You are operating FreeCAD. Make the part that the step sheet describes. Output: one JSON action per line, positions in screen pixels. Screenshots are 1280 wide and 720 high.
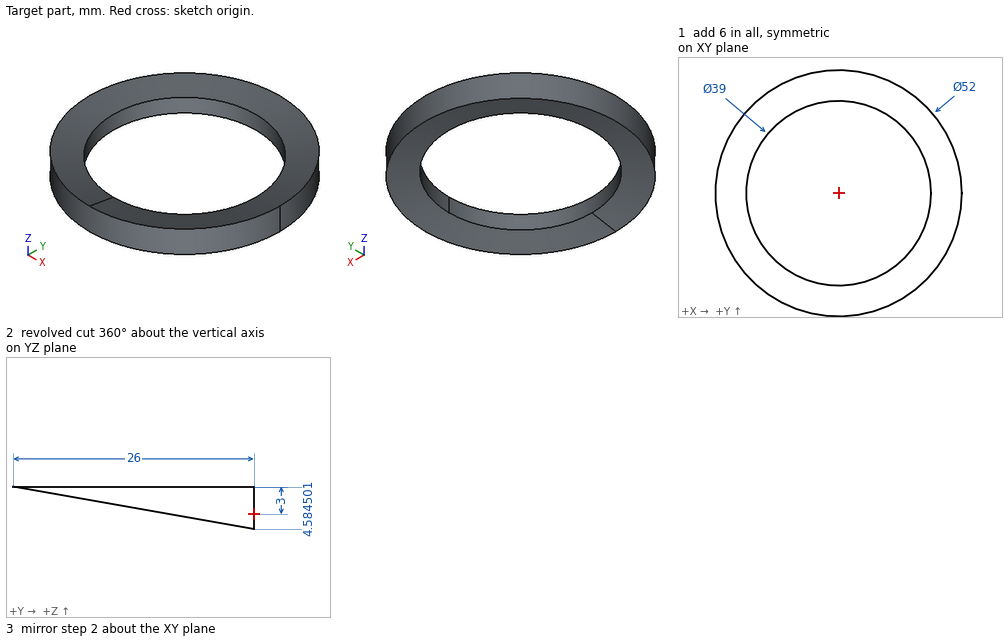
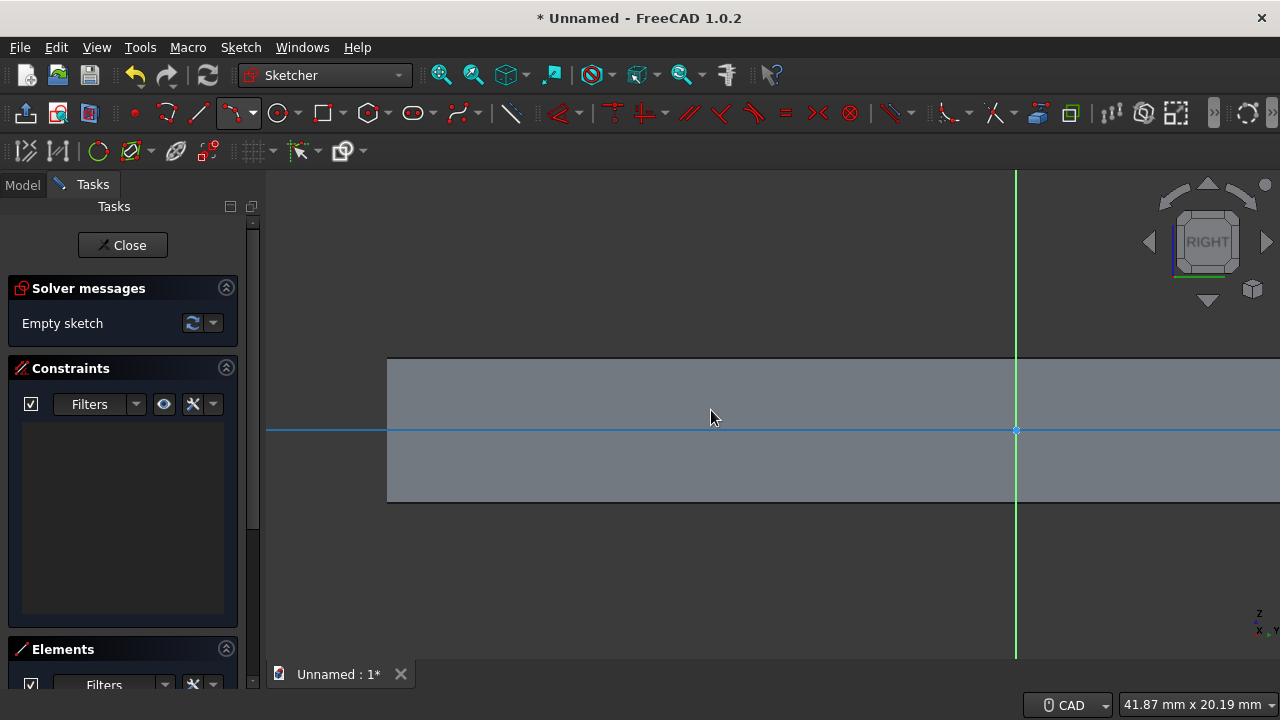
{"action": "key", "text": "g m"}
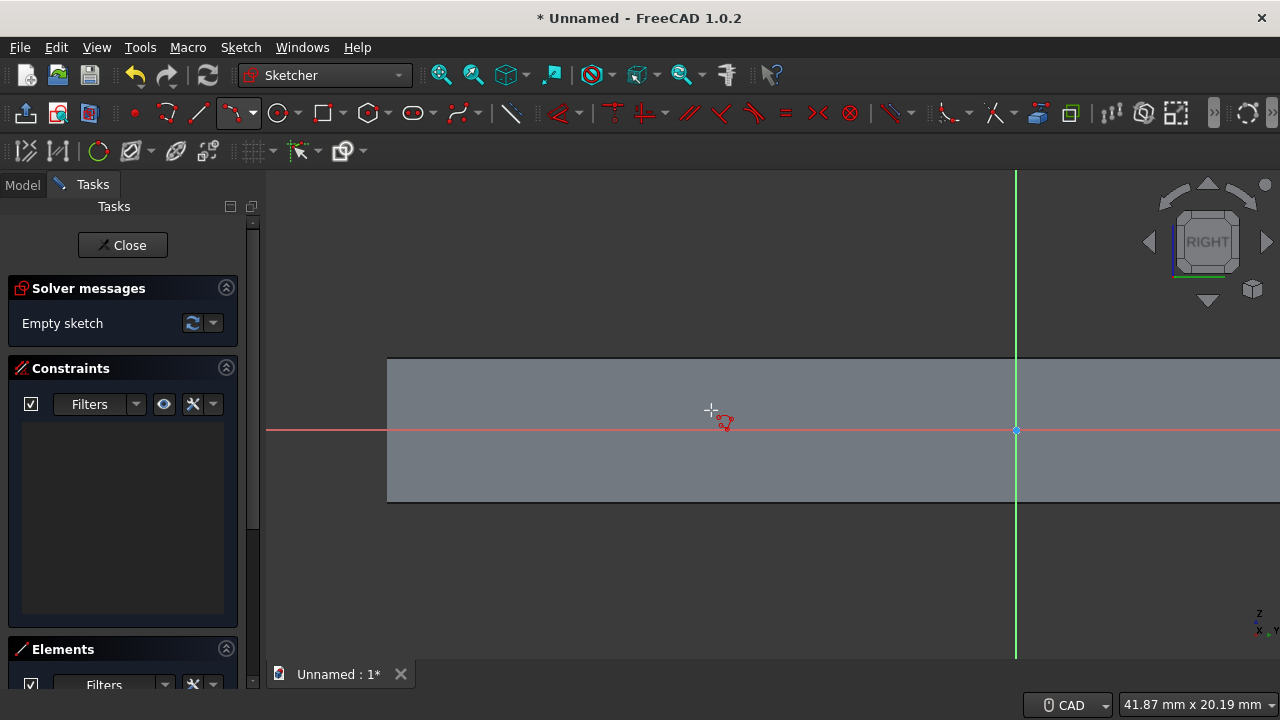
{"action": "left_click", "coordinate": [1016, 469]}
{"action": "left_click", "coordinate": [1007, 358]}
{"action": "left_click", "coordinate": [387, 358]}
{"action": "left_click", "coordinate": [1016, 470]}
{"action": "key", "text": "Escape"}
{"action": "key", "text": "Escape"}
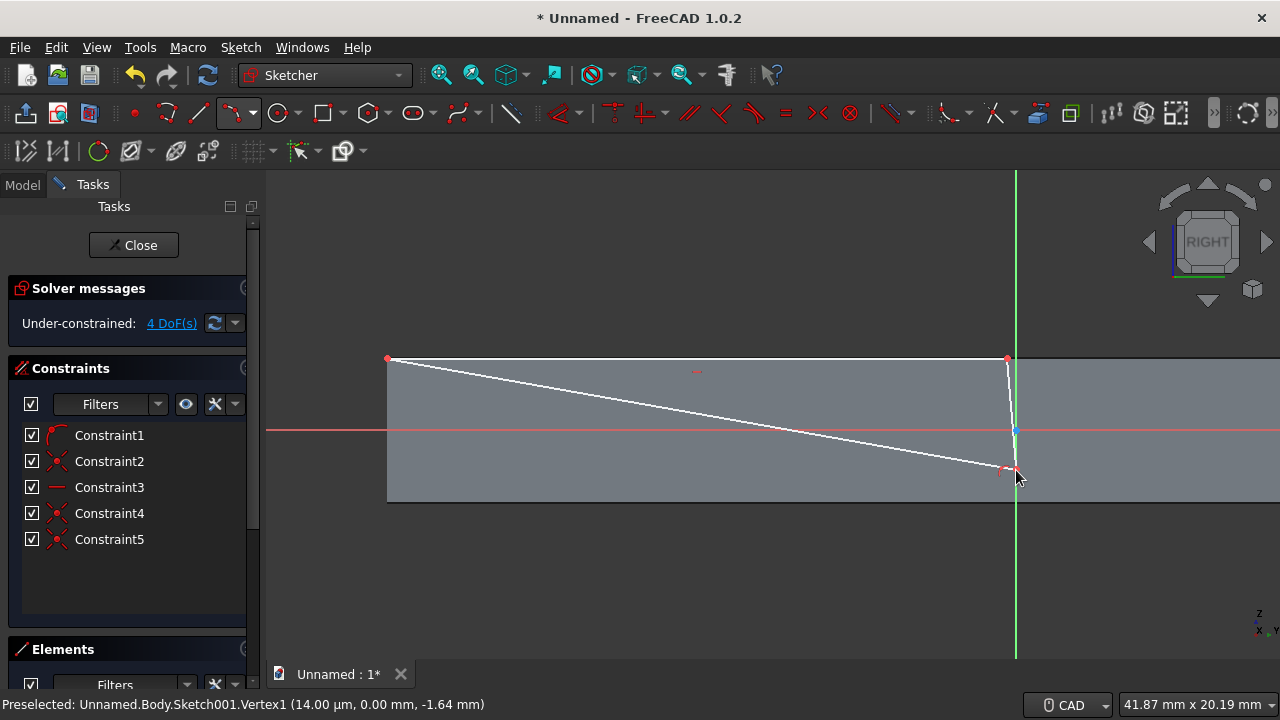
{"action": "left_click", "coordinate": [1014, 448]}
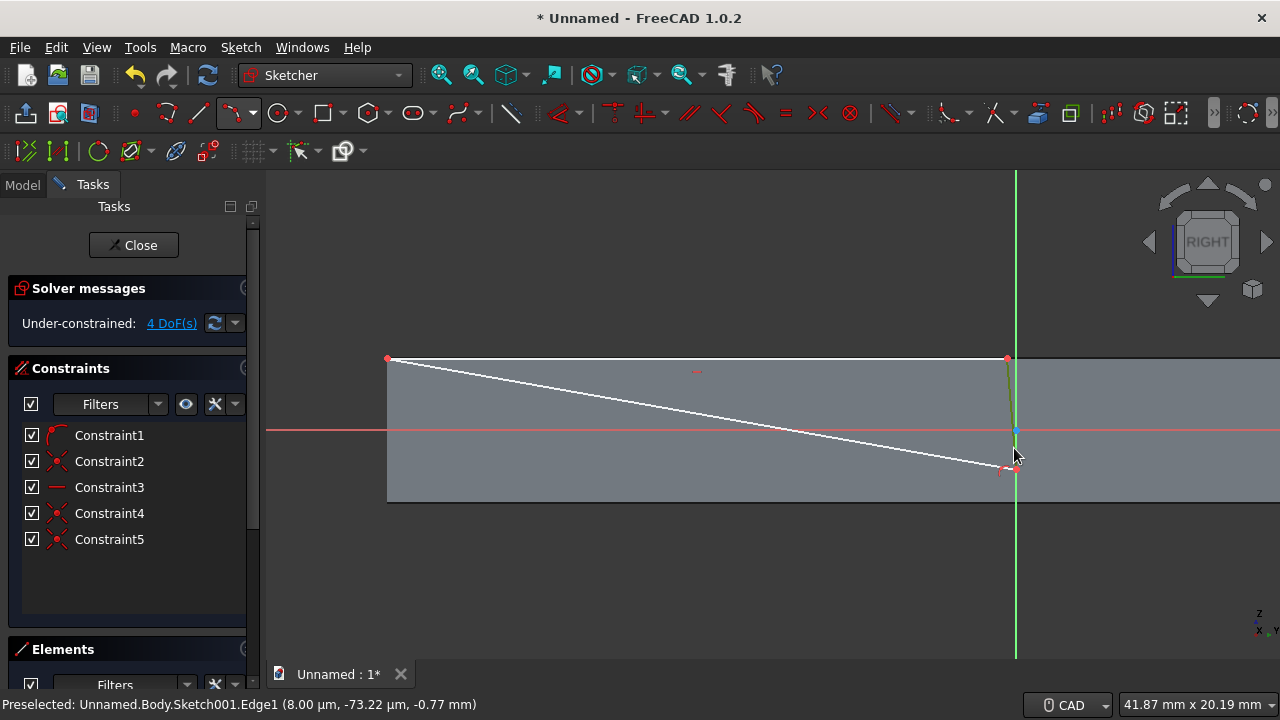
{"action": "key", "text": "v"}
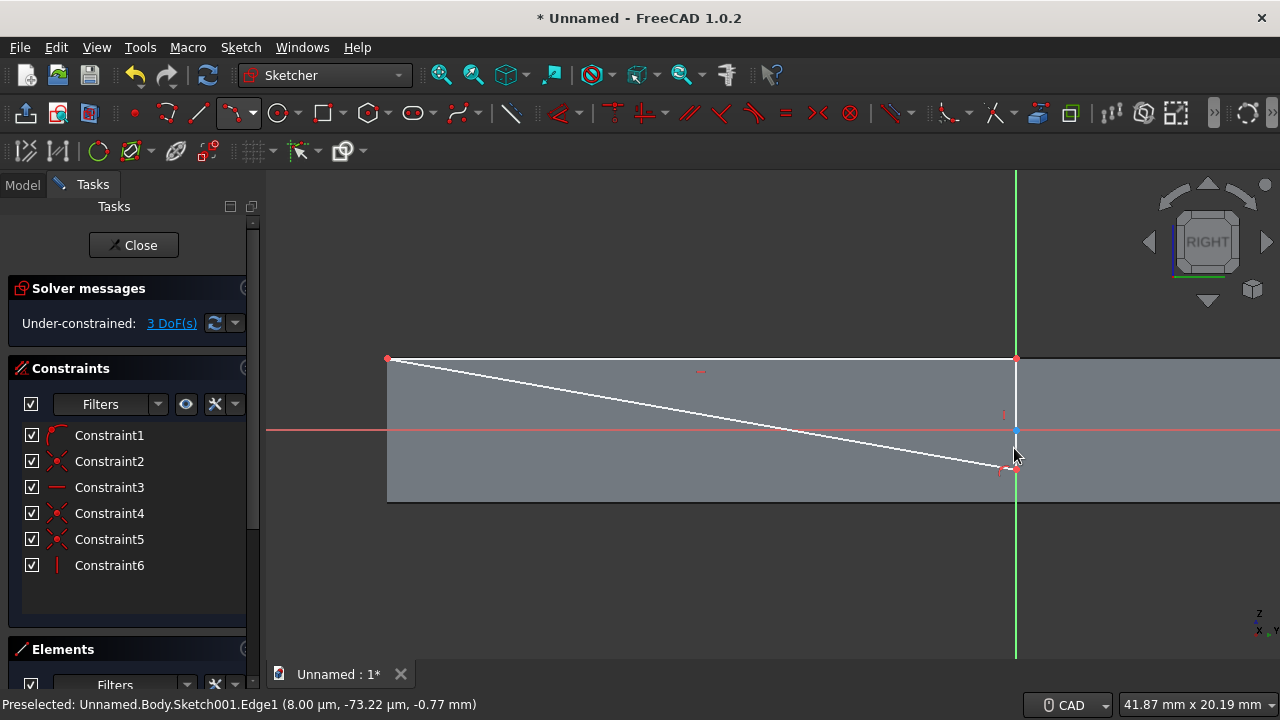
{"action": "left_click", "coordinate": [558, 114]}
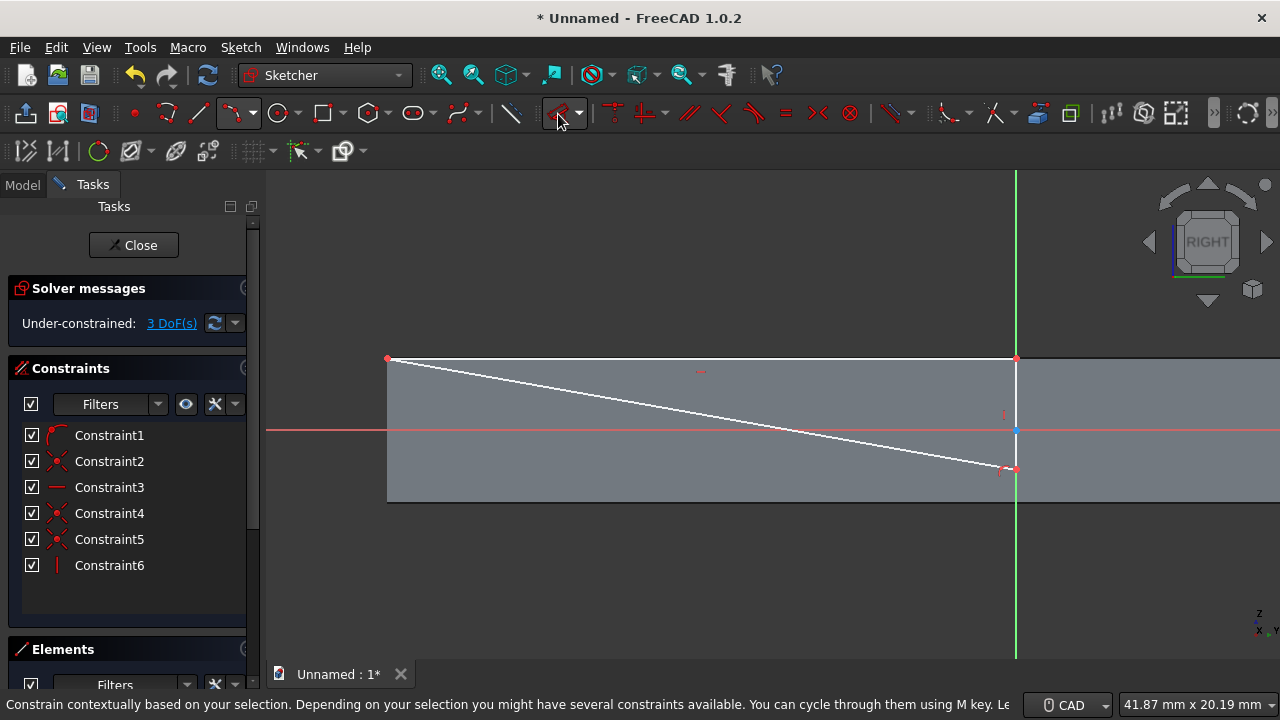
{"action": "left_click", "coordinate": [828, 359]}
{"action": "left_click", "coordinate": [702, 325]}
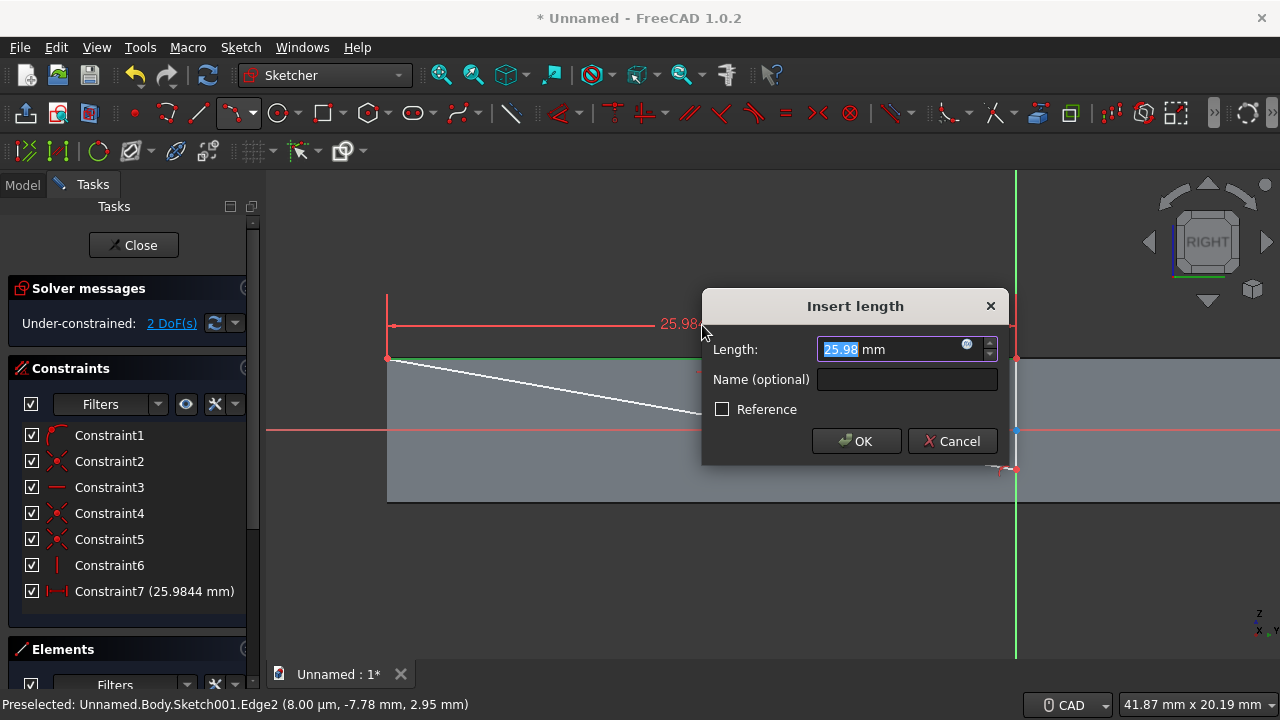
{"action": "type", "text": "26"}
{"action": "key", "text": "Return"}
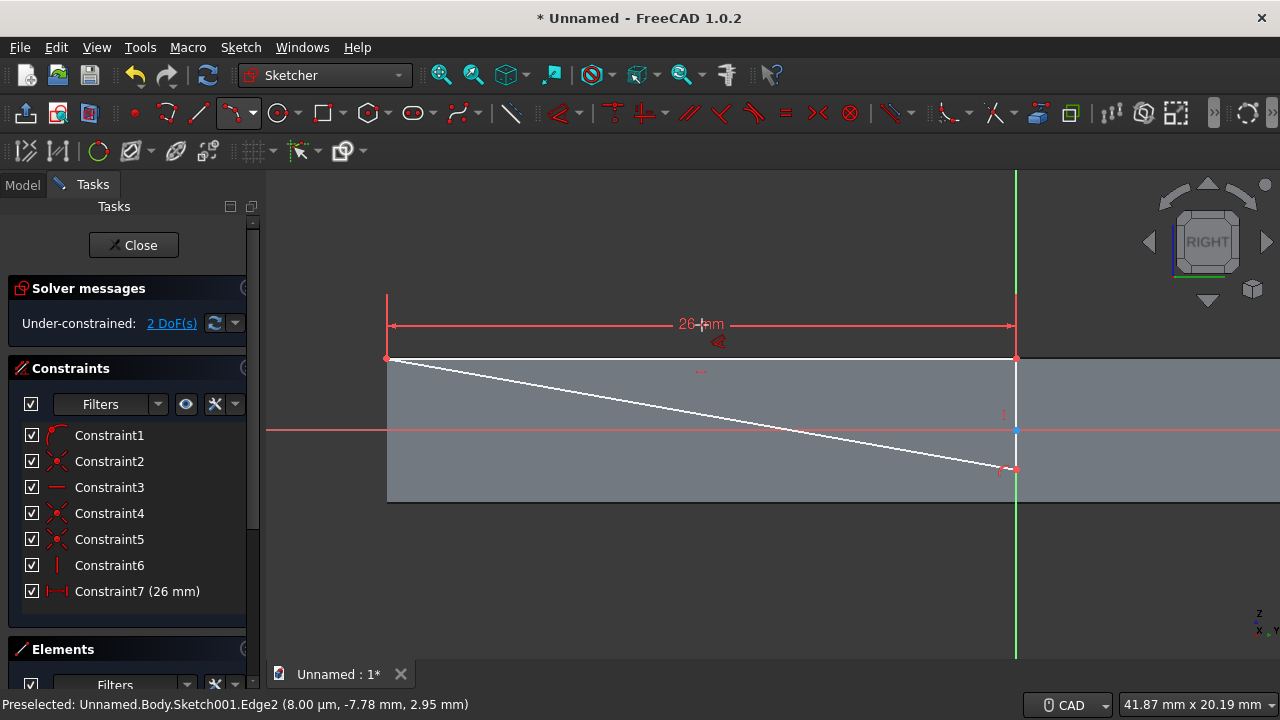
{"action": "left_click", "coordinate": [1016, 359]}
{"action": "left_click", "coordinate": [1050, 395]}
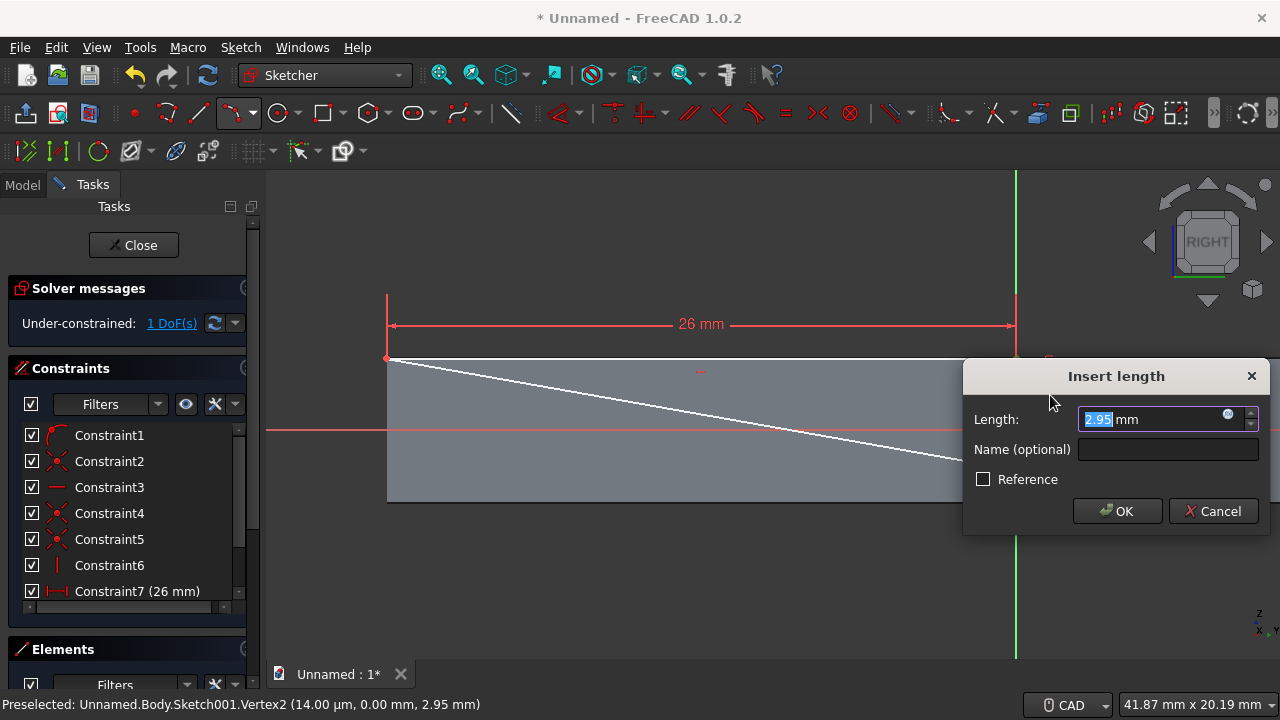
{"action": "type", "text": "3"}
{"action": "key", "text": "Return"}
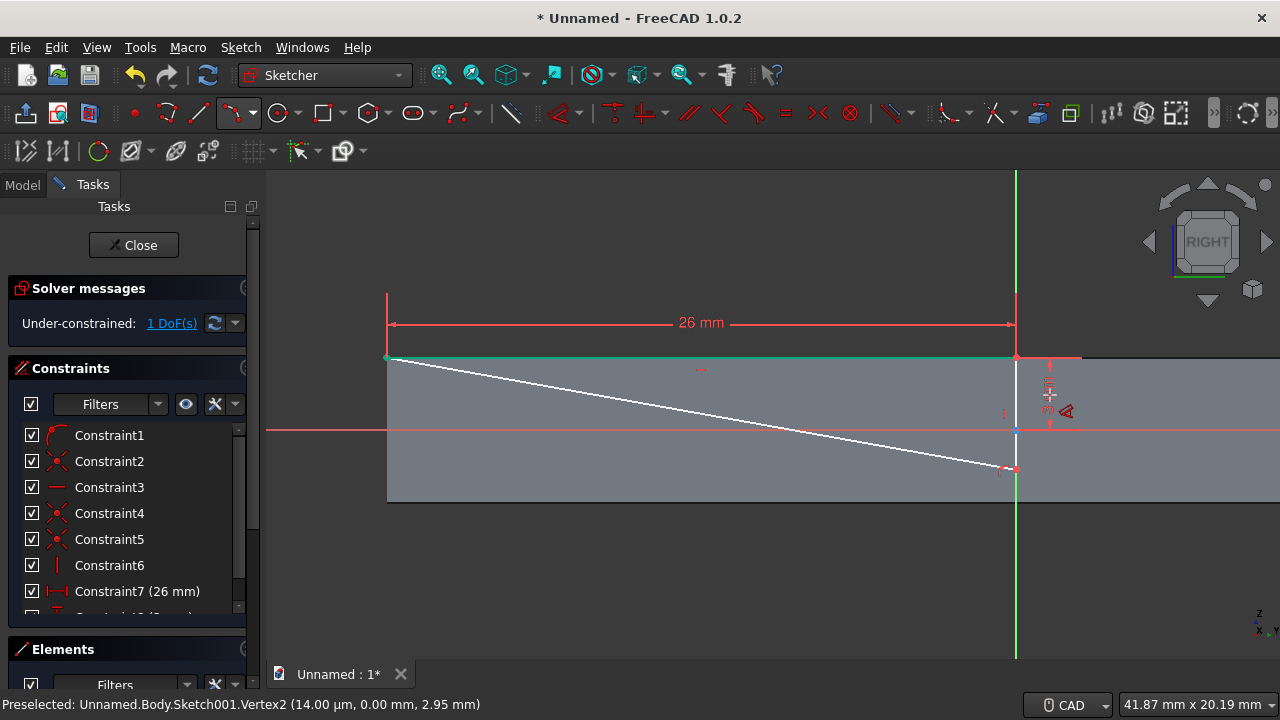
{"action": "left_click", "coordinate": [1016, 391]}
{"action": "left_click", "coordinate": [1050, 375]}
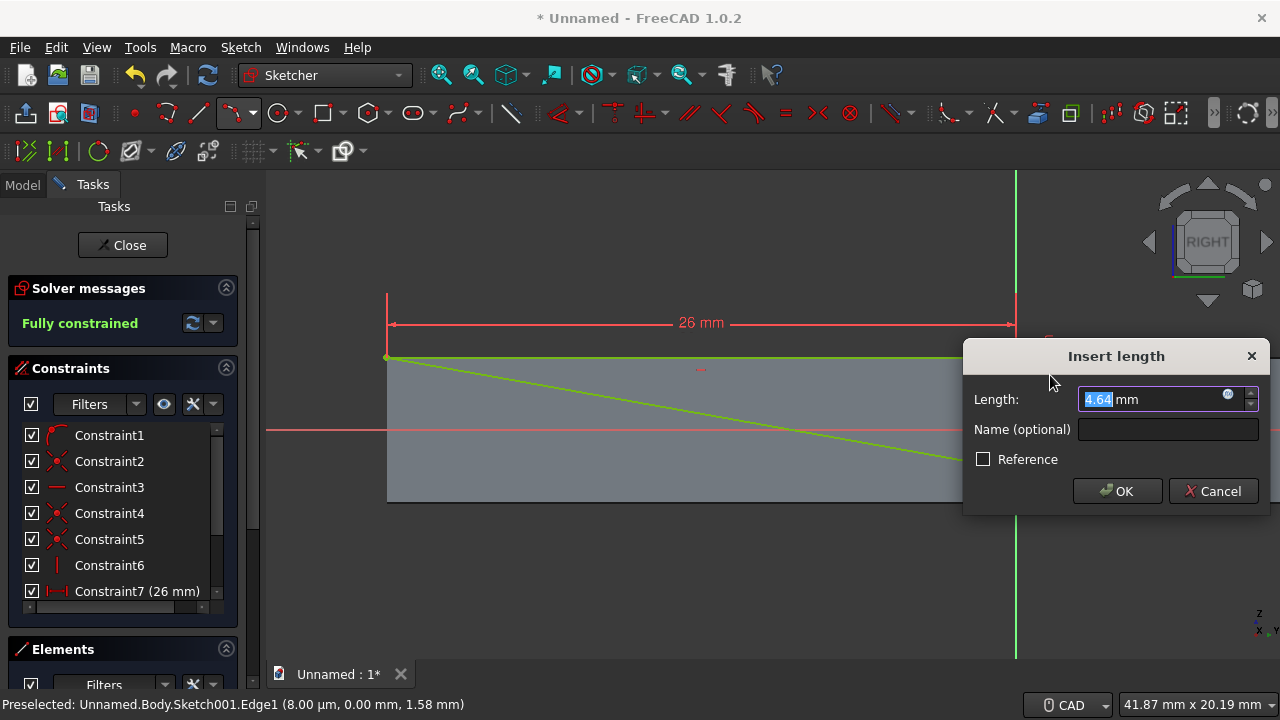
{"action": "type", "text": "4.584501"}
{"action": "key", "text": "Return"}
{"action": "key", "text": "Escape"}